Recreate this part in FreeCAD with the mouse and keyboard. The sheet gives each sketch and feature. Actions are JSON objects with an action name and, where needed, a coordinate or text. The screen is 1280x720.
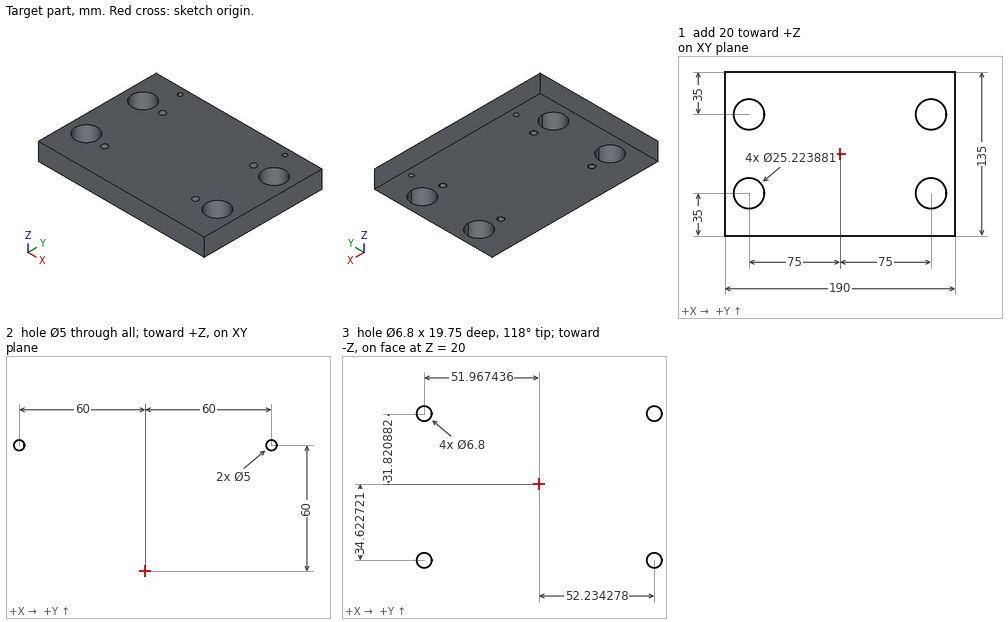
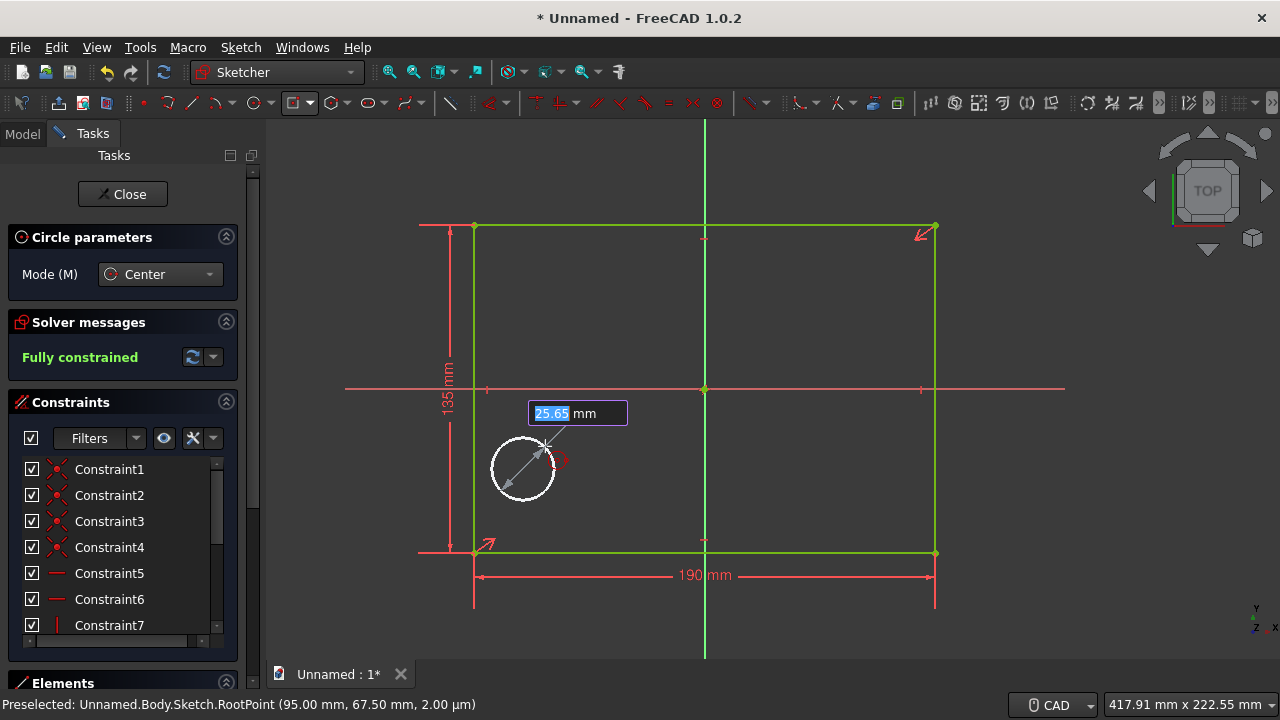
{"action": "type", "text": "25.223881"}
{"action": "key", "text": "Return"}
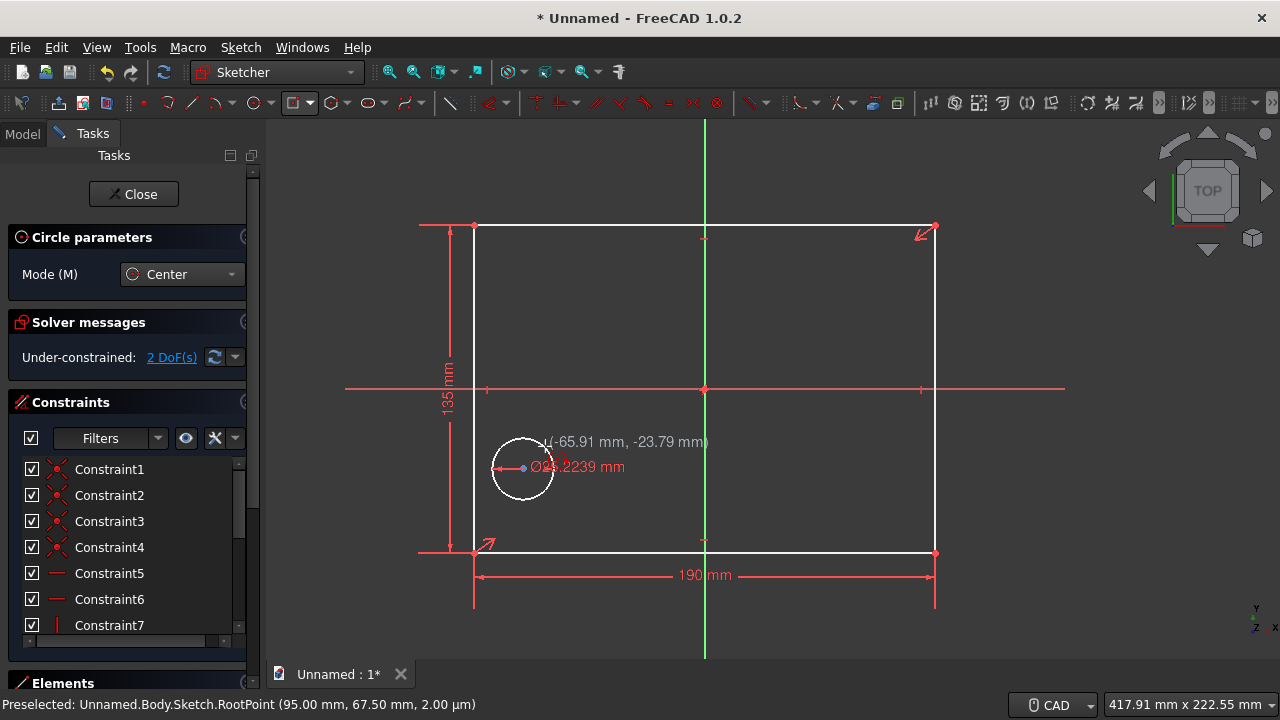
{"action": "left_click", "coordinate": [887, 468]}
{"action": "mouse_move", "coordinate": [909, 446]}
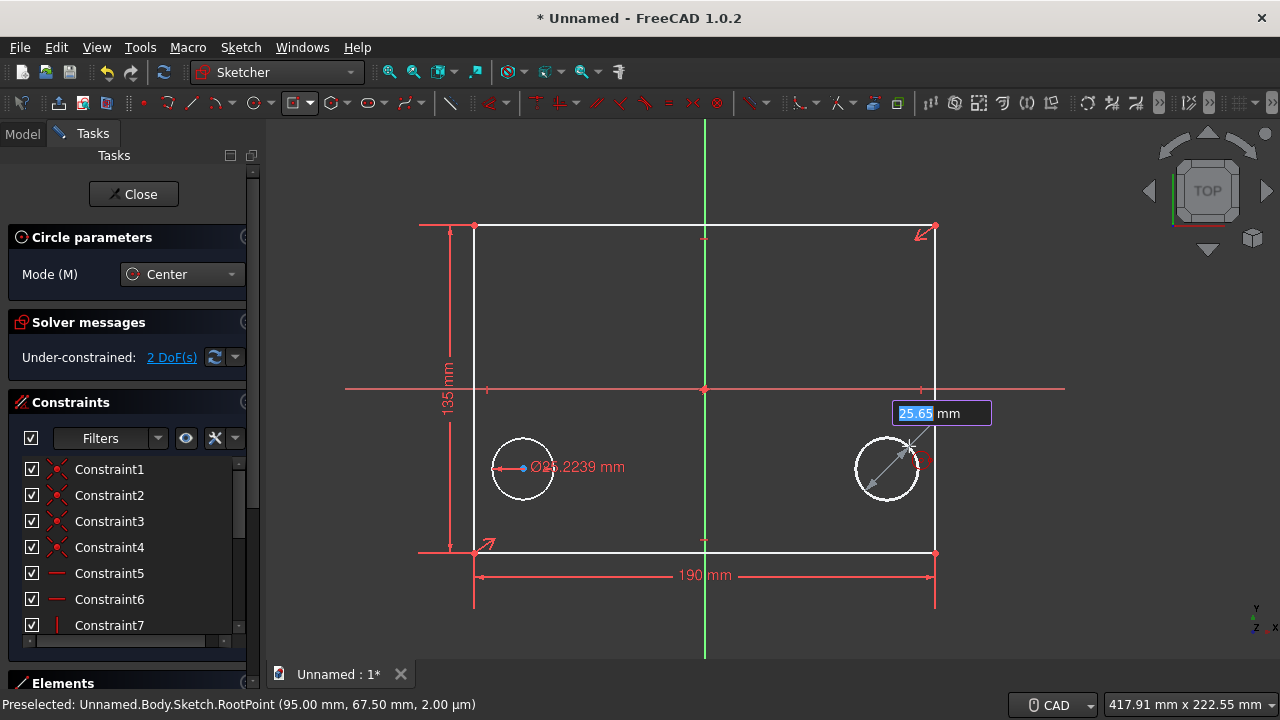
{"action": "type", "text": "25.223881"}
{"action": "key", "text": "Return"}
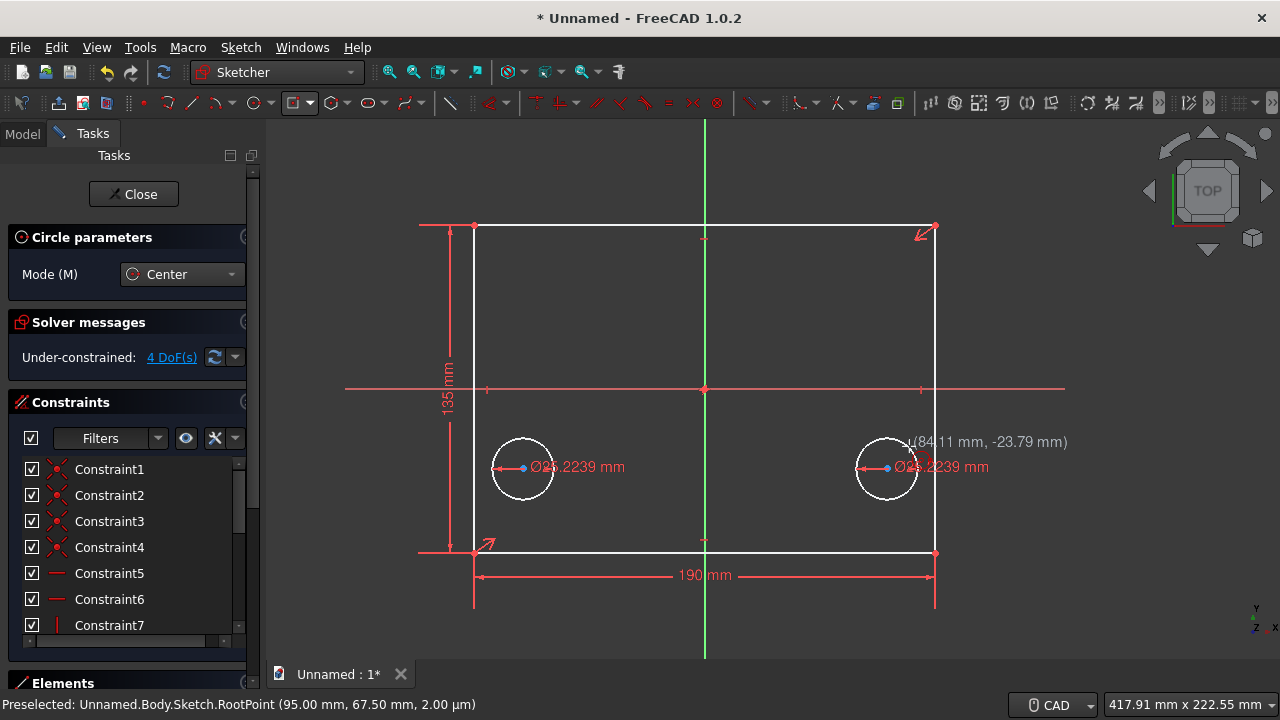
{"action": "left_click", "coordinate": [523, 310]}
{"action": "mouse_move", "coordinate": [545, 289]}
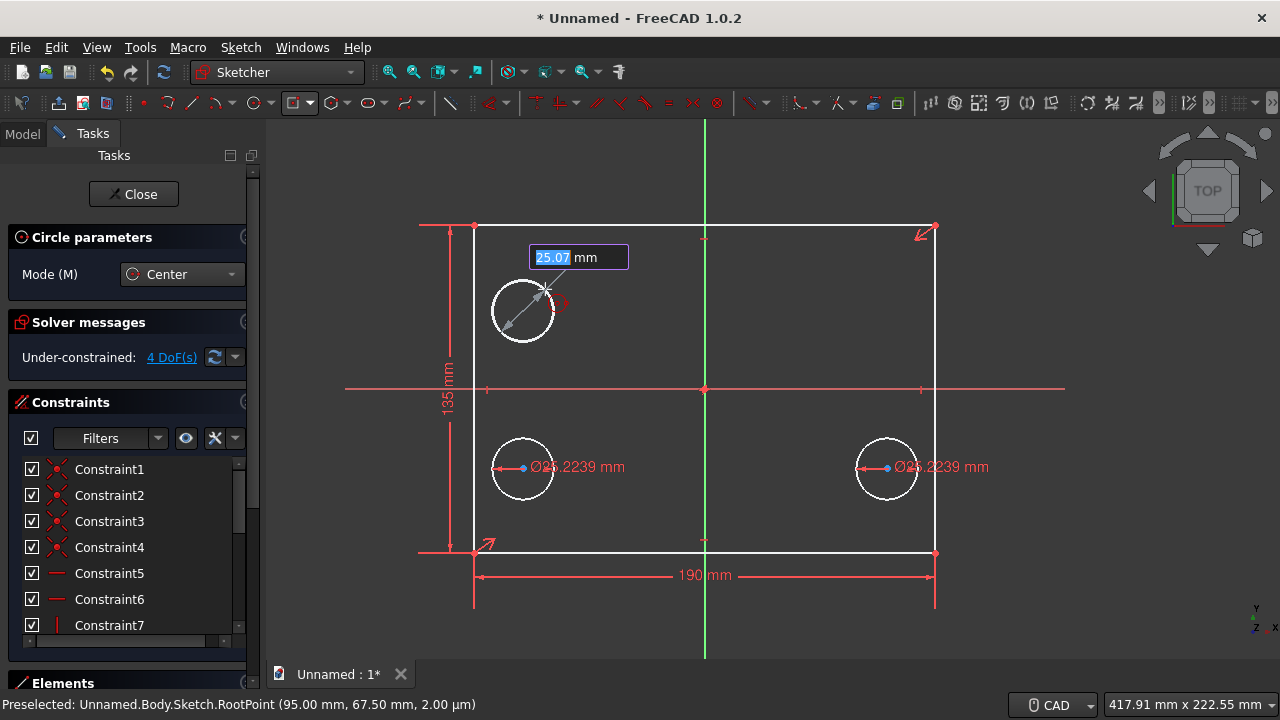
{"action": "type", "text": "25.223881"}
{"action": "key", "text": "Return"}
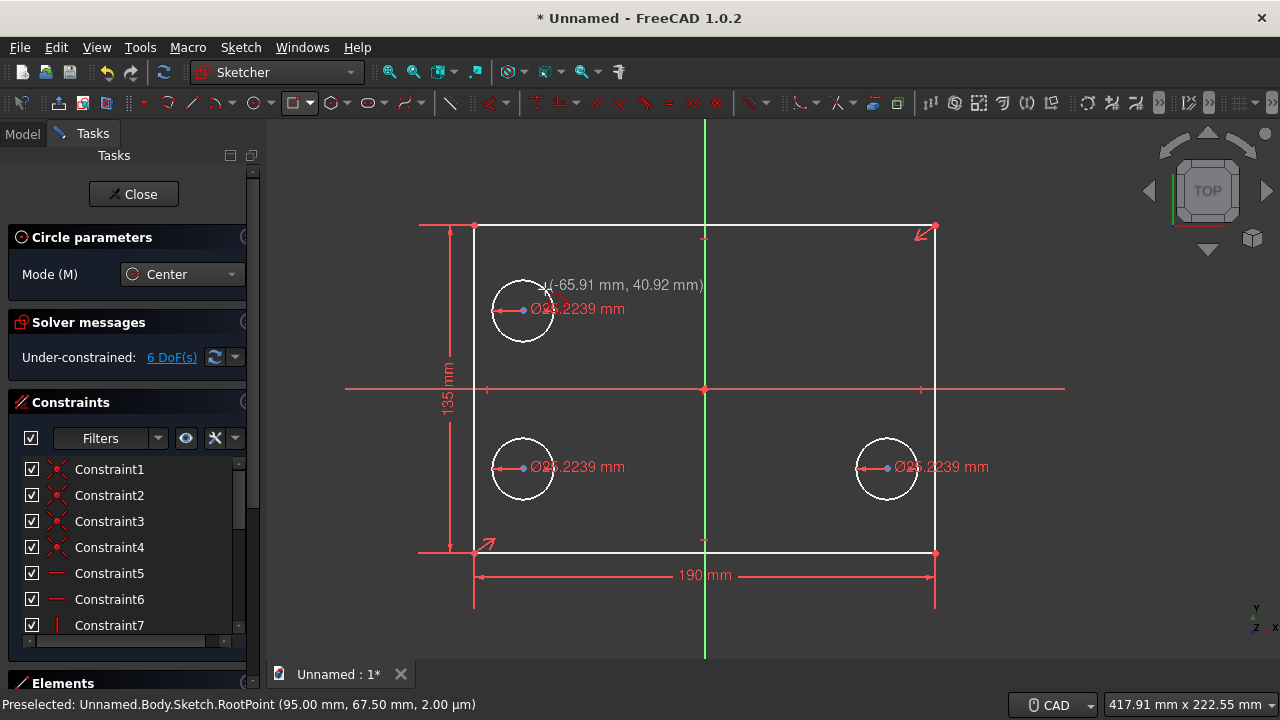
{"action": "left_click", "coordinate": [887, 310]}
{"action": "mouse_move", "coordinate": [909, 289]}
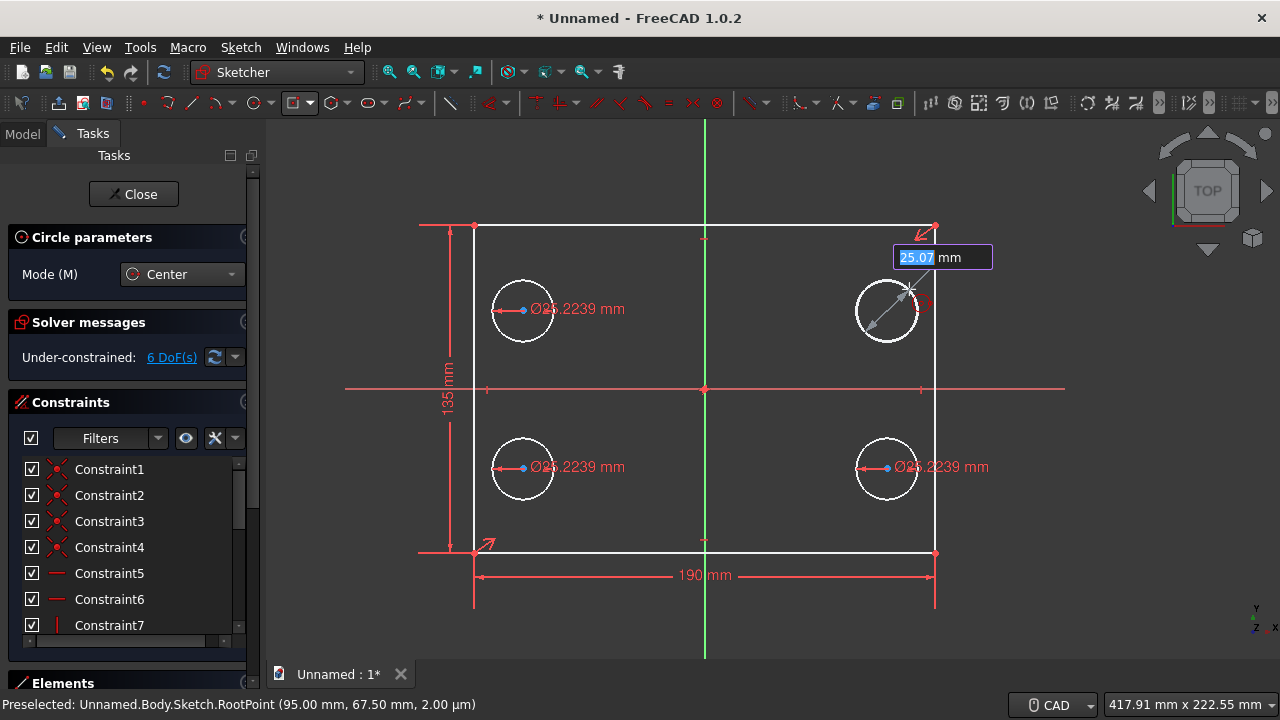
{"action": "type", "text": "25.223881"}
{"action": "key", "text": "Return"}
{"action": "key", "text": "Escape"}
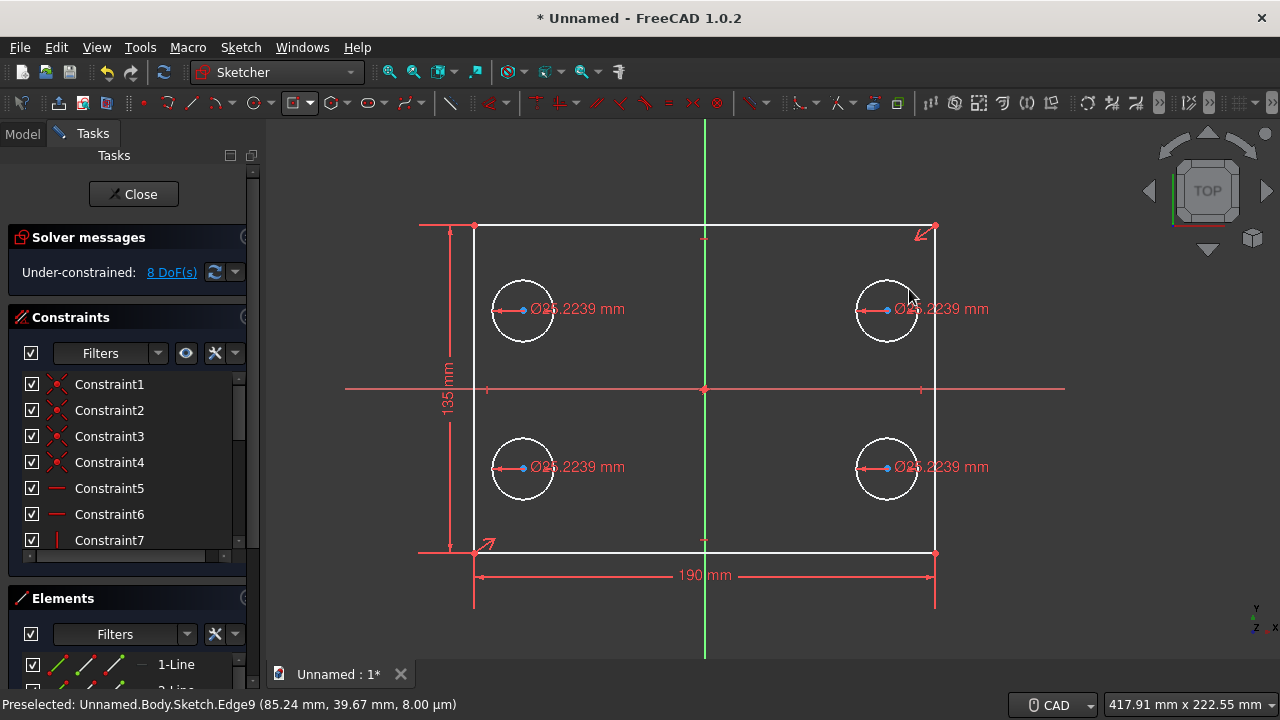
{"action": "left_click", "coordinate": [523, 469]}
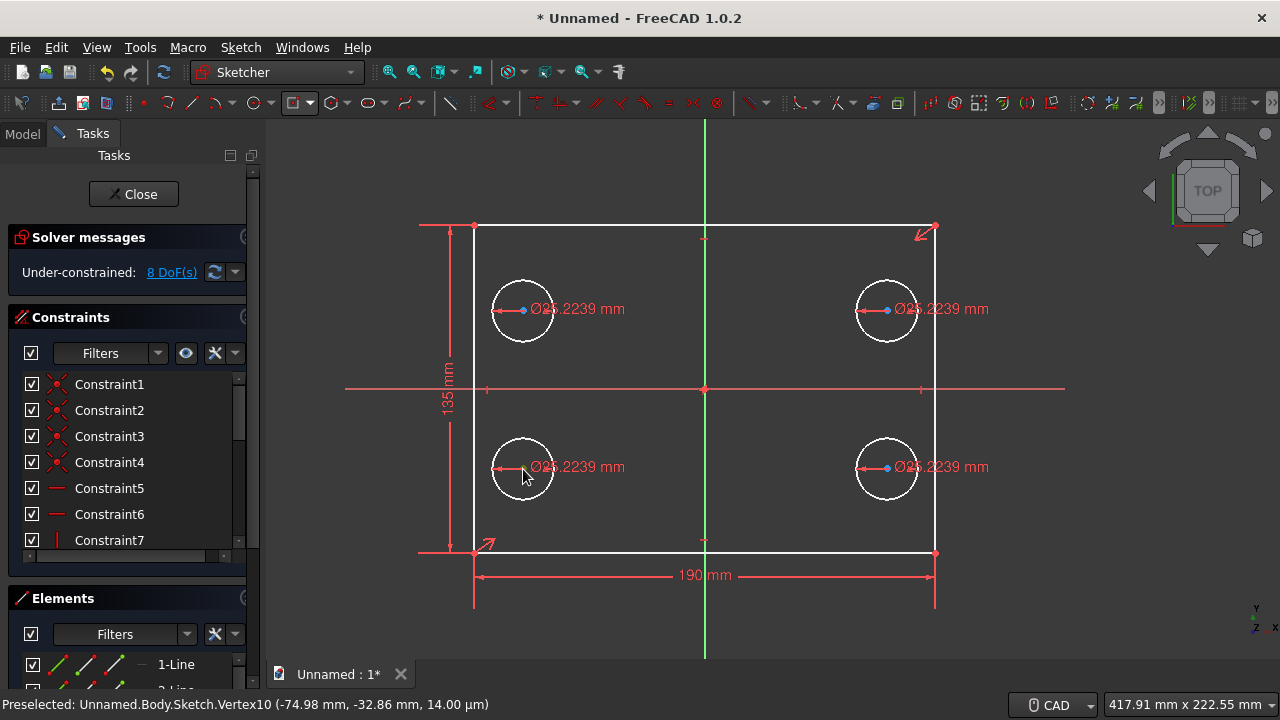
{"action": "left_click", "coordinate": [887, 469]}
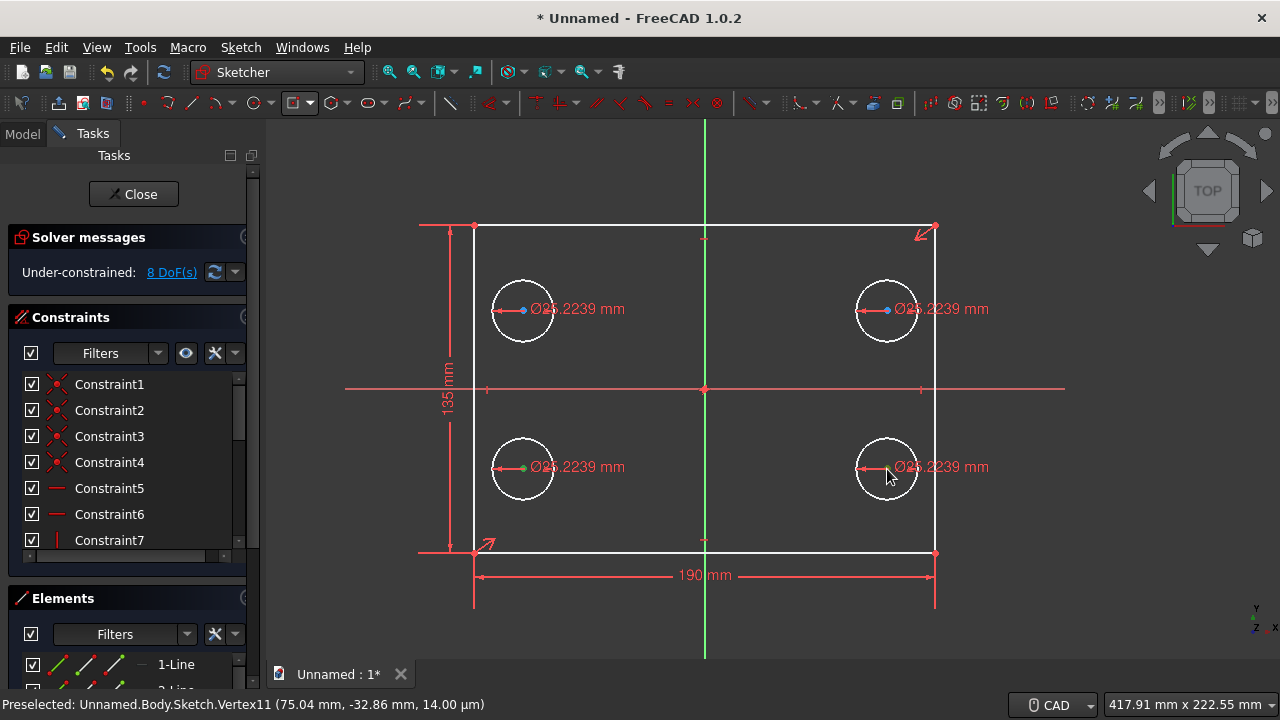
{"action": "key", "text": "h"}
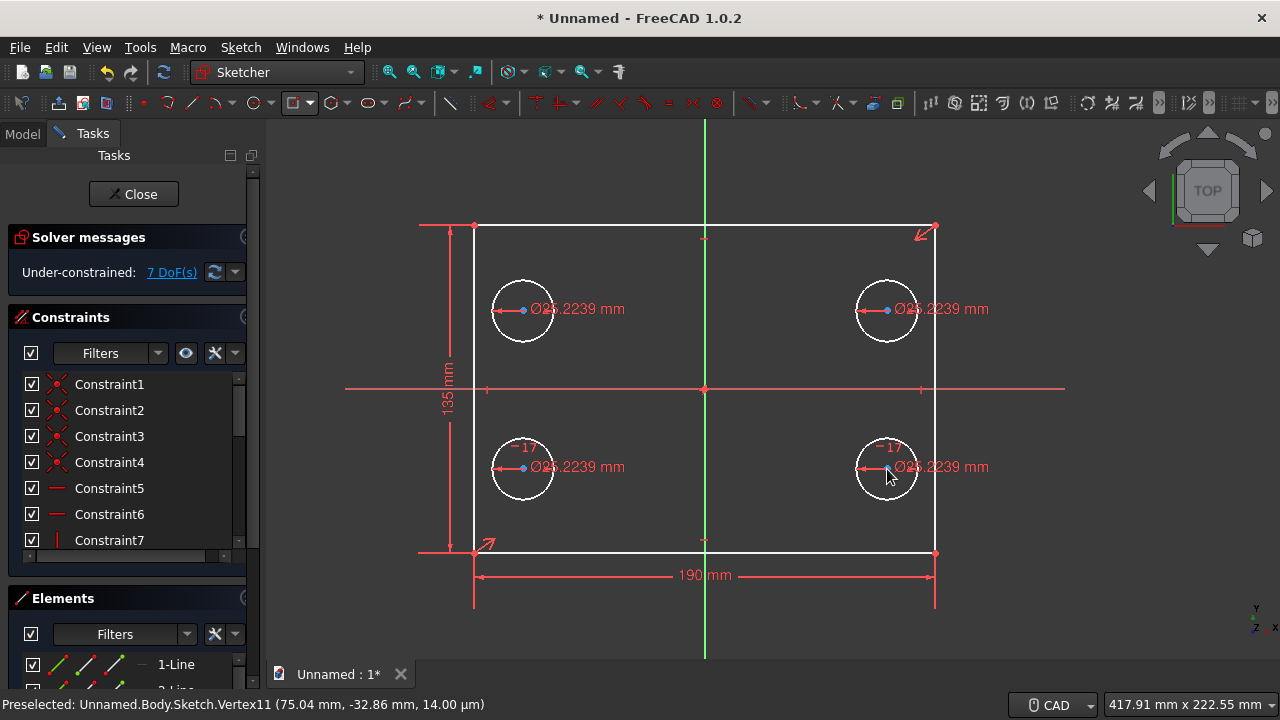
{"action": "left_click", "coordinate": [523, 469]}